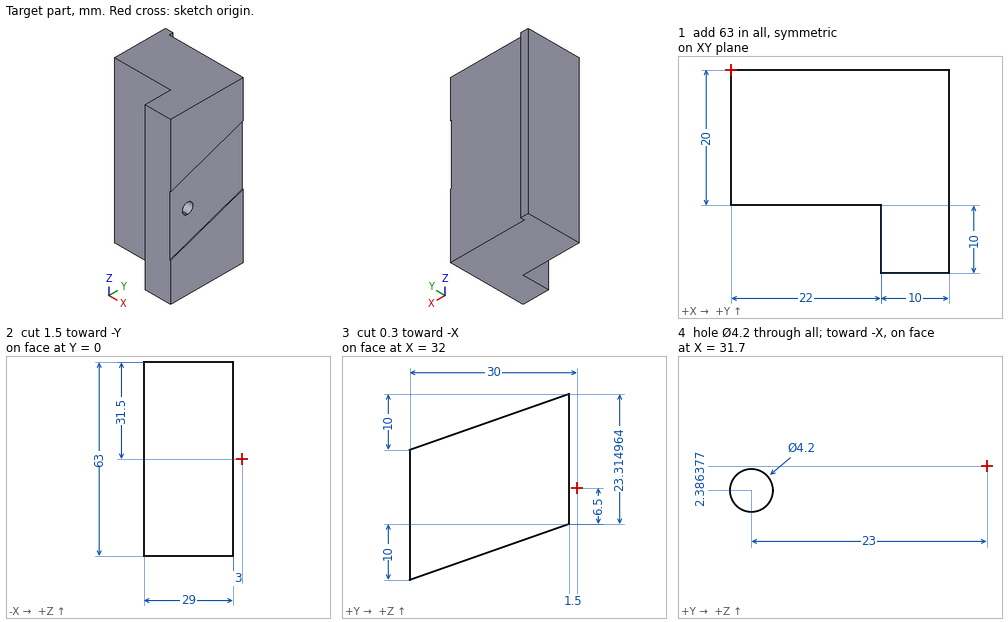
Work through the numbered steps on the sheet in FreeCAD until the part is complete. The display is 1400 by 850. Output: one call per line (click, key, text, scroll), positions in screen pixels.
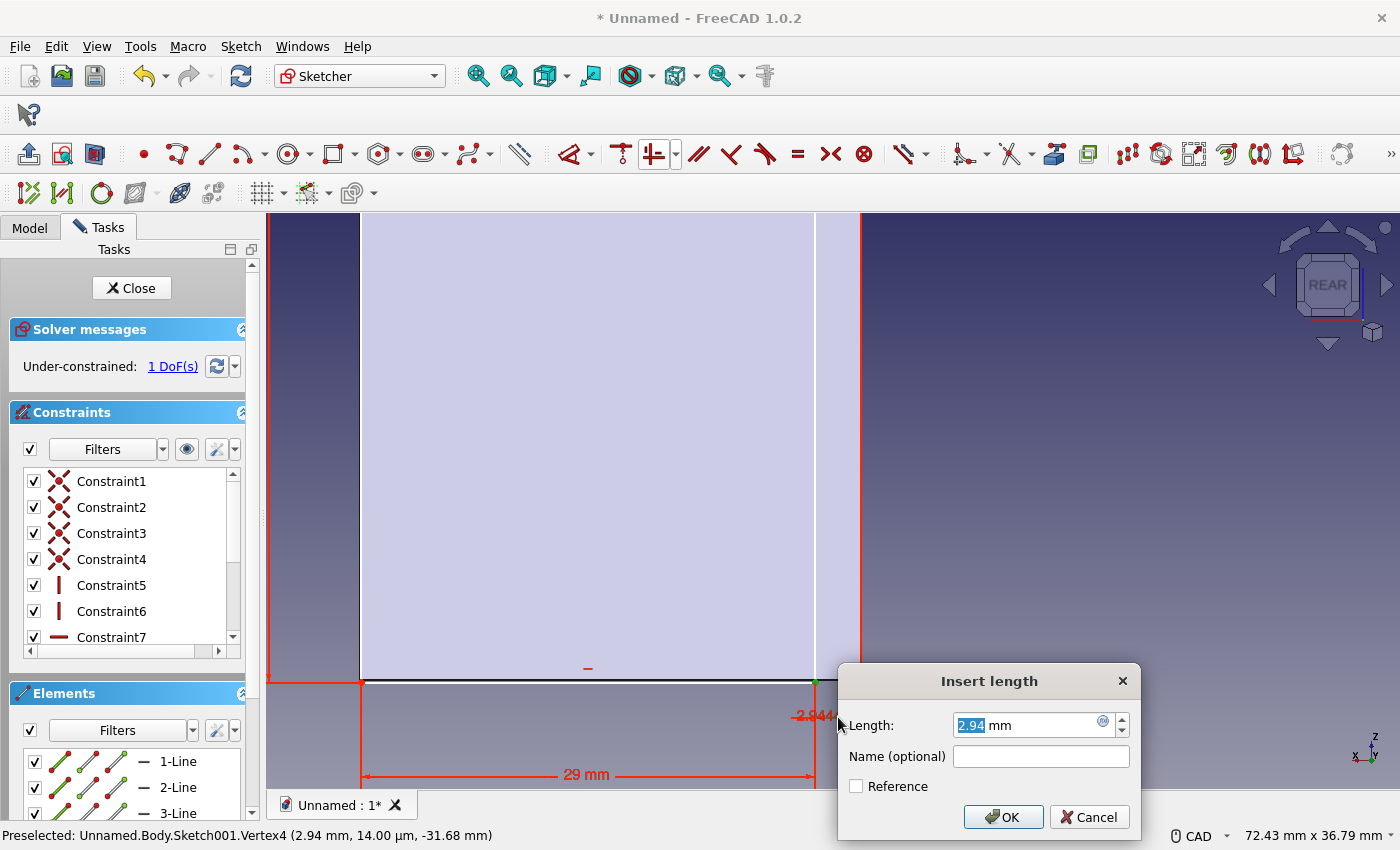
text(3)
key(Return)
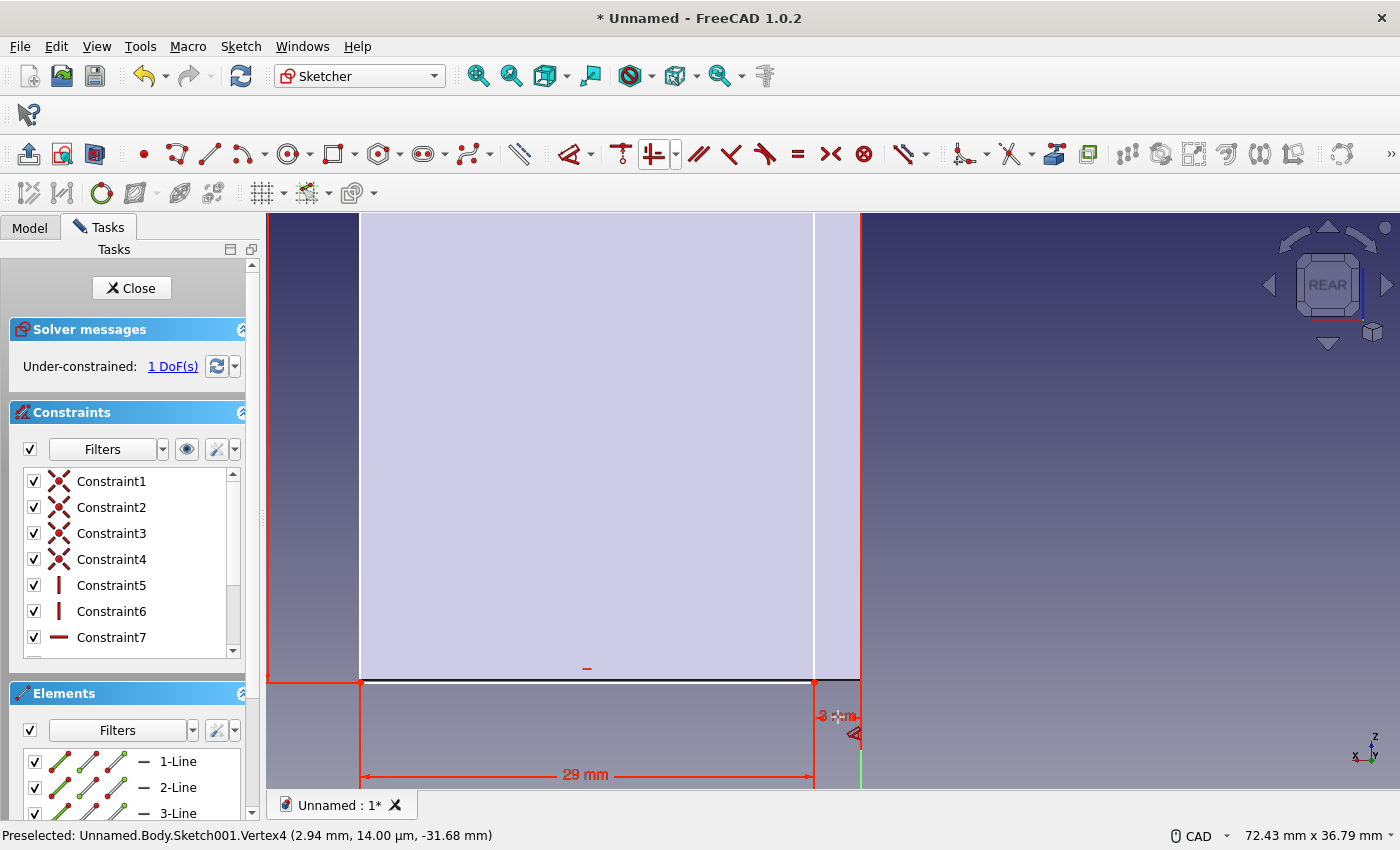
scroll(854, 684, down, 5)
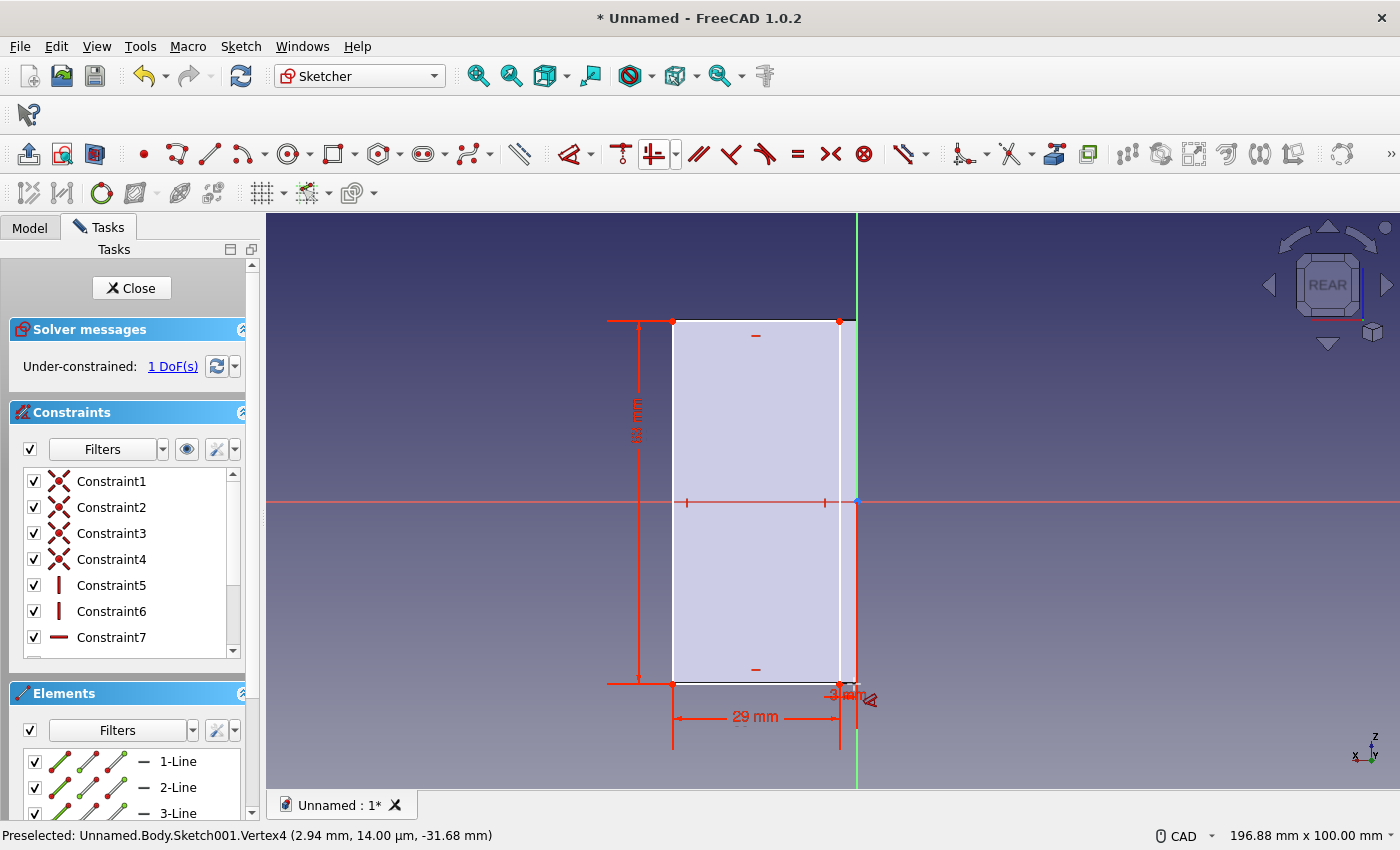
click(673, 321)
click(891, 411)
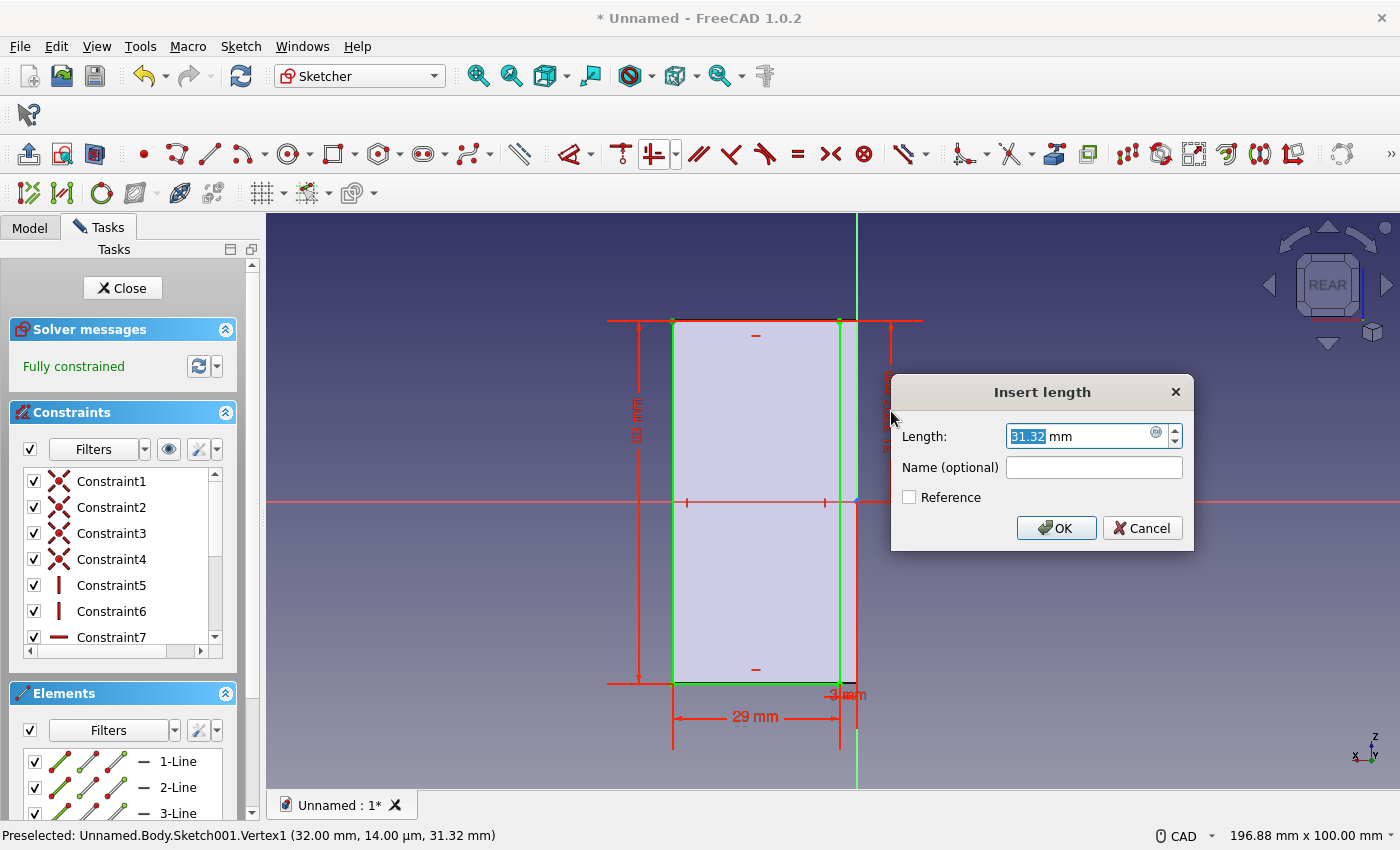
text(31.5)
key(Return)
key(Escape)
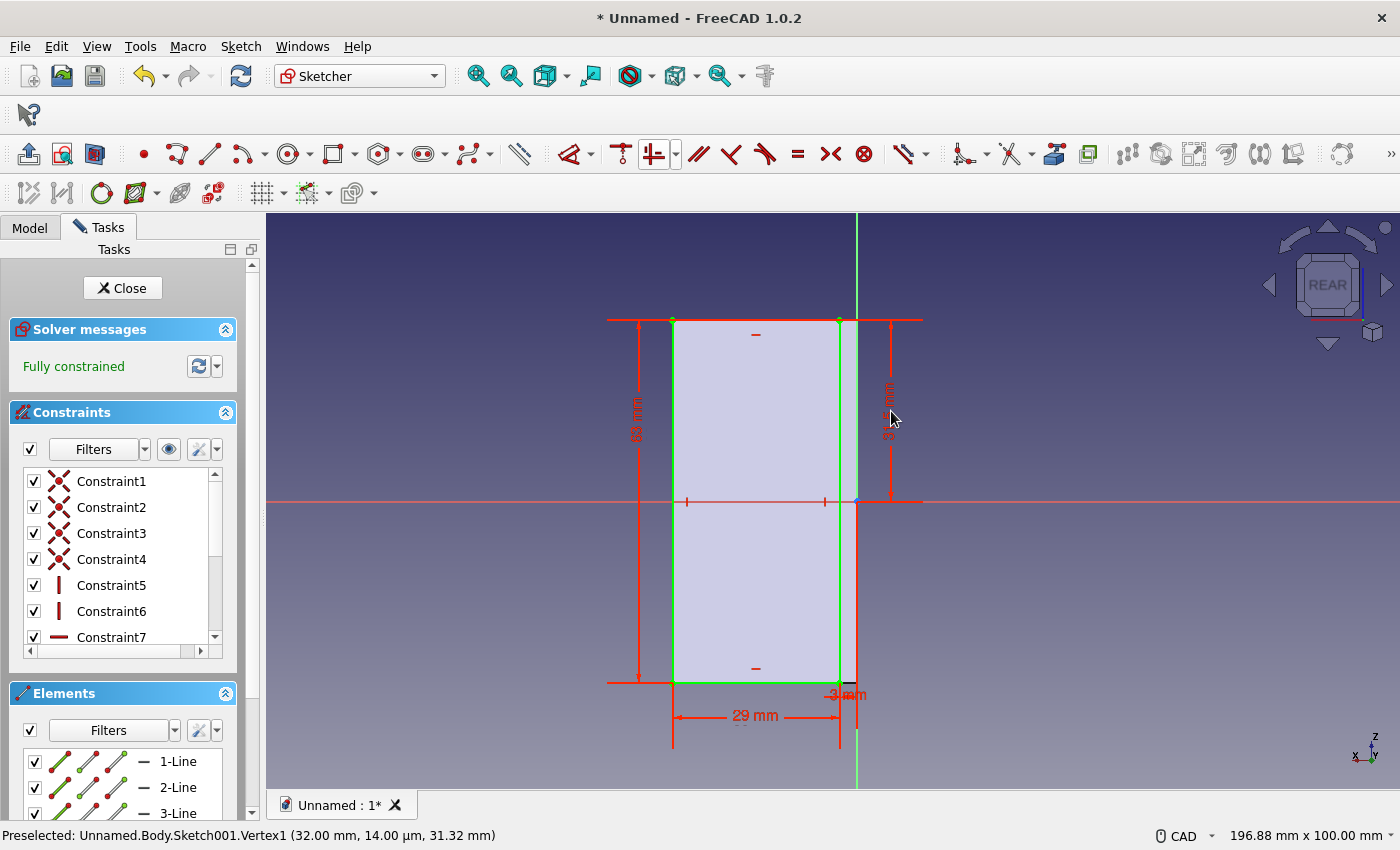
click(123, 288)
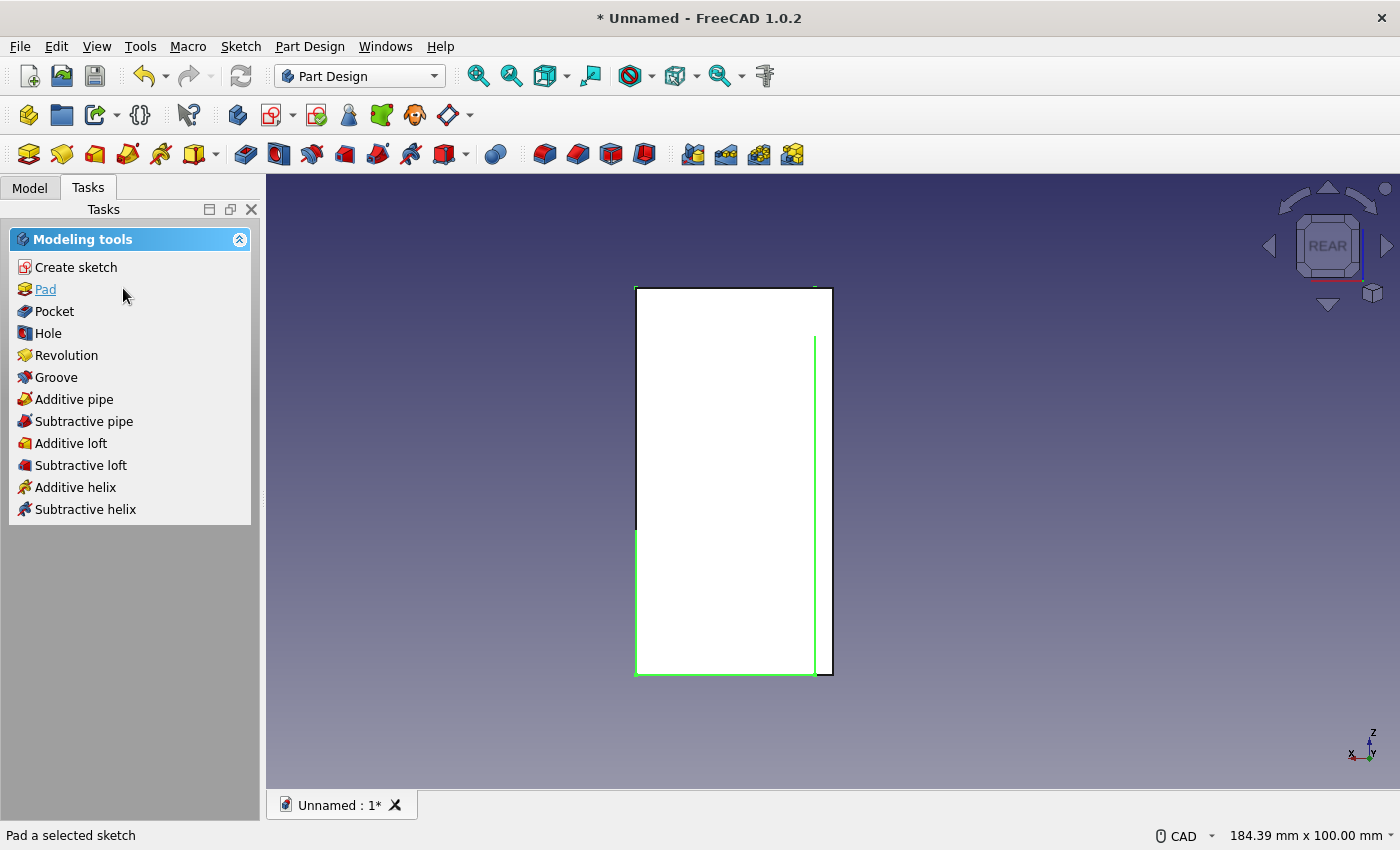
click(246, 154)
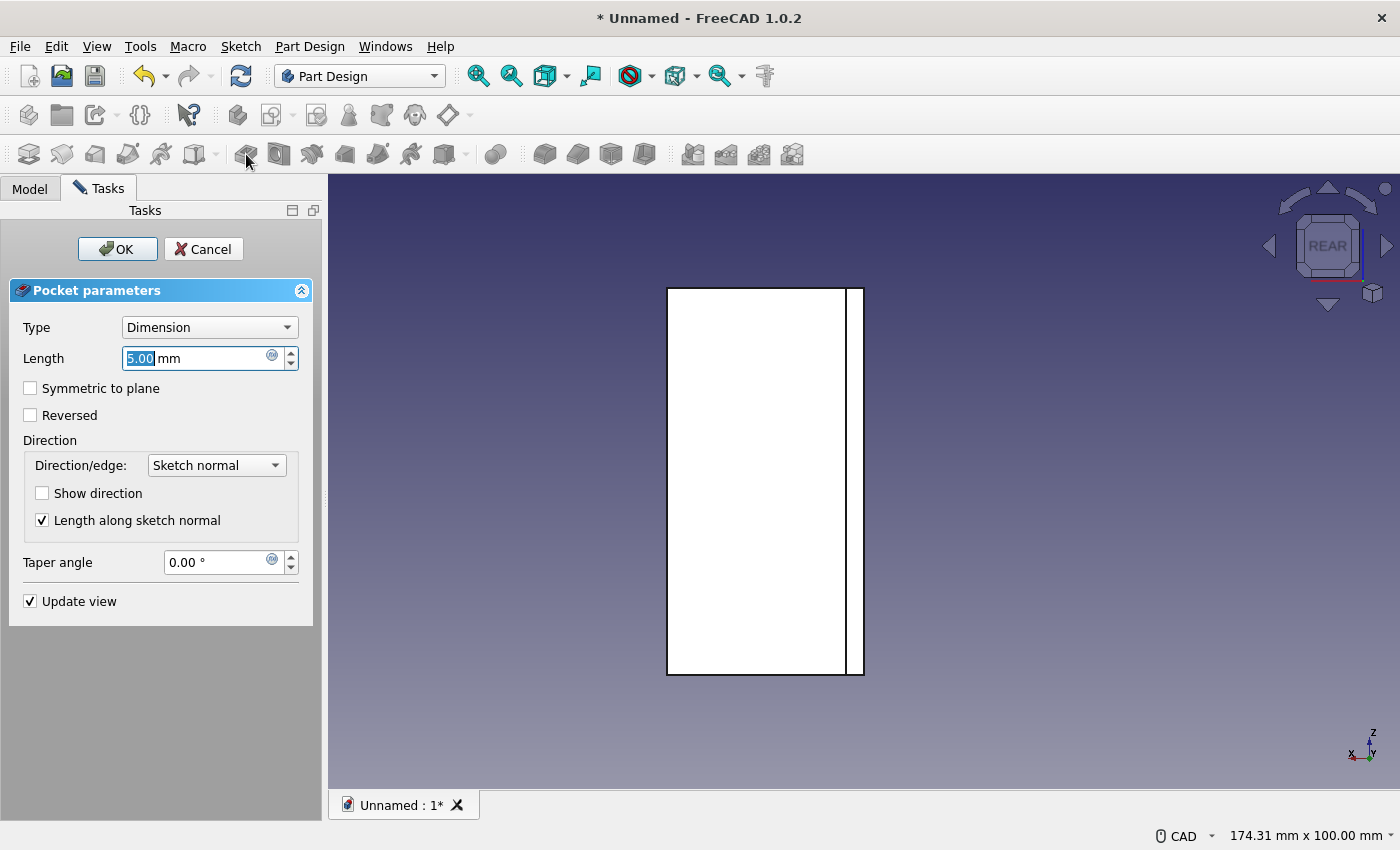
text(1.5)
key(Tab)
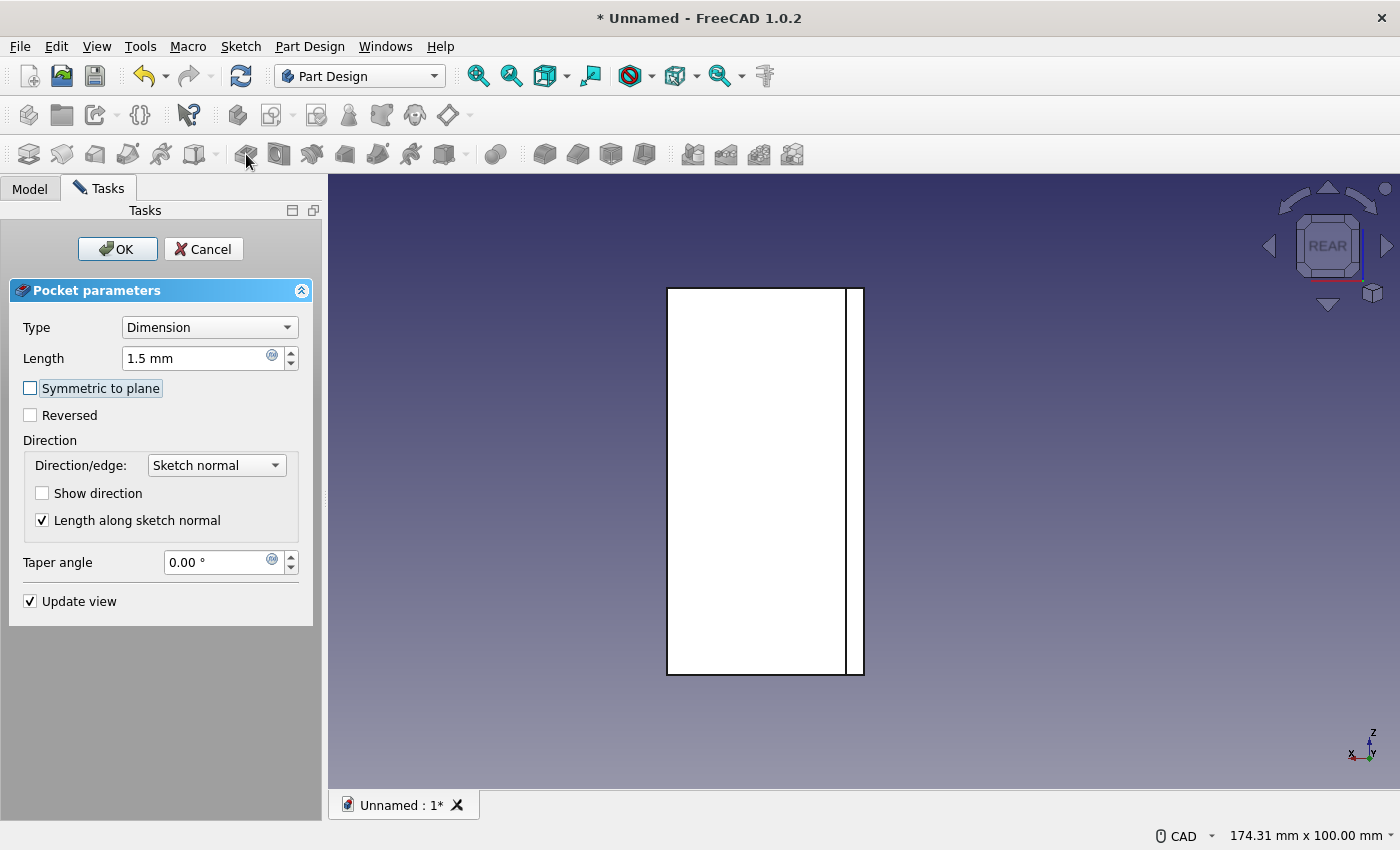
click(118, 249)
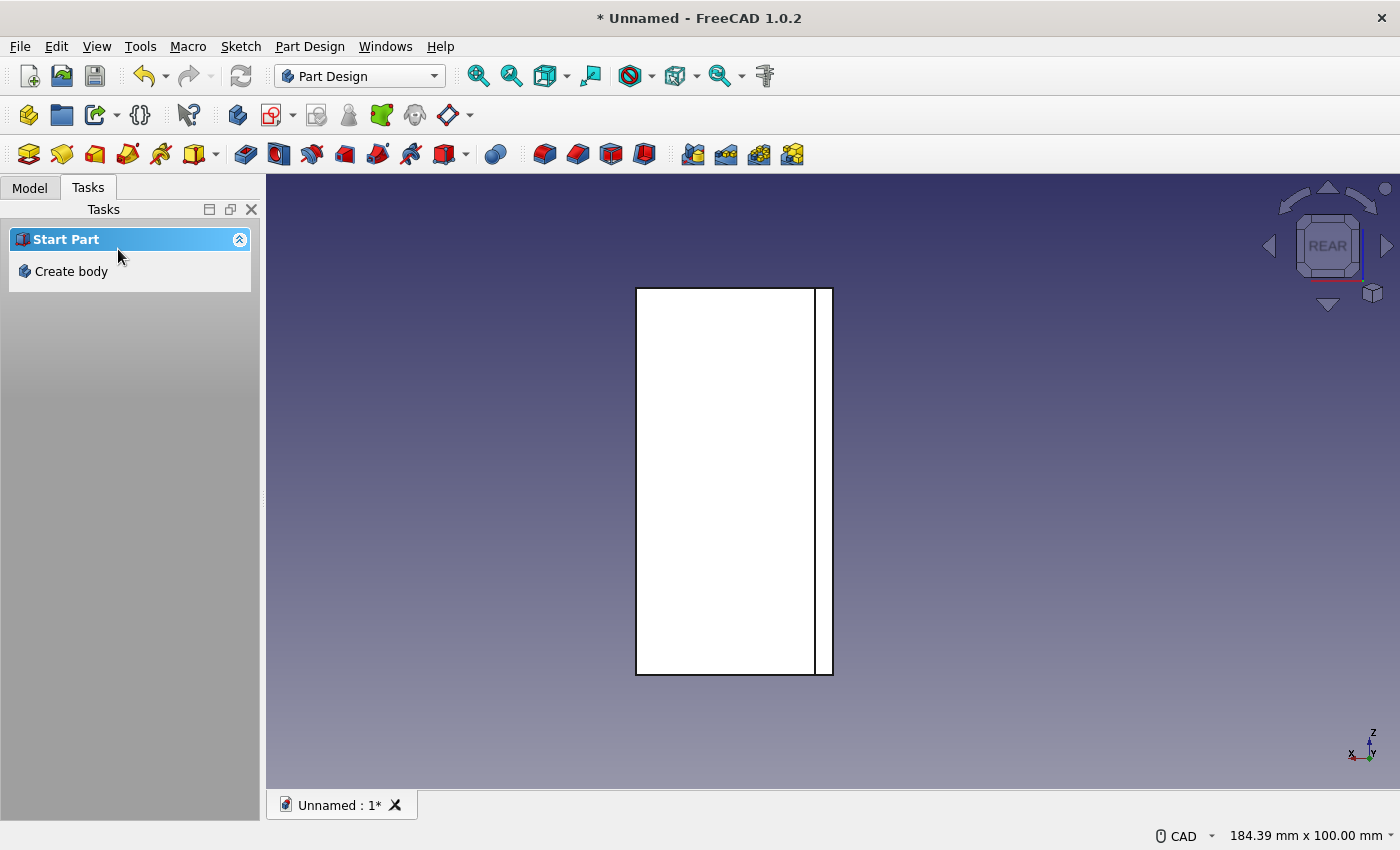
key(0)